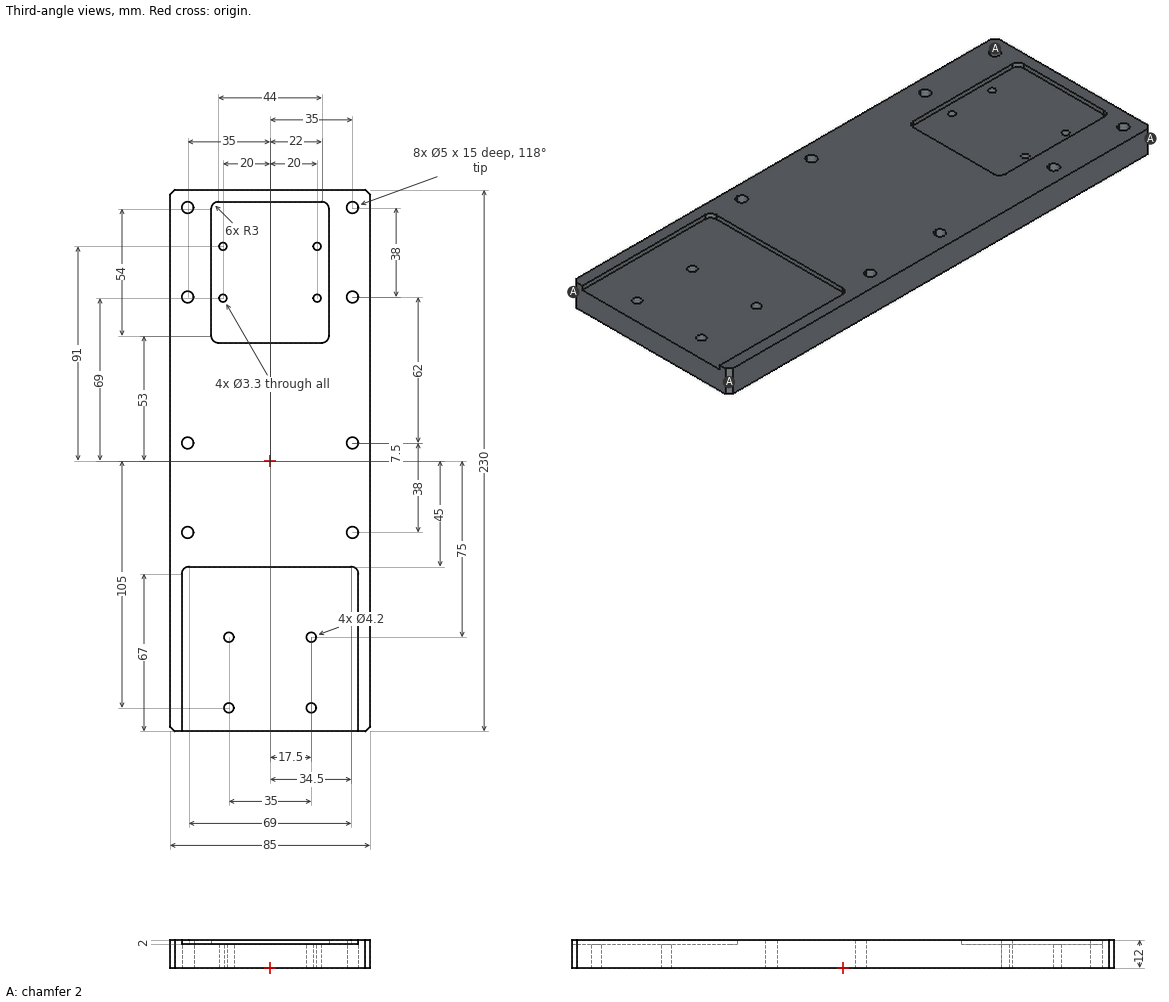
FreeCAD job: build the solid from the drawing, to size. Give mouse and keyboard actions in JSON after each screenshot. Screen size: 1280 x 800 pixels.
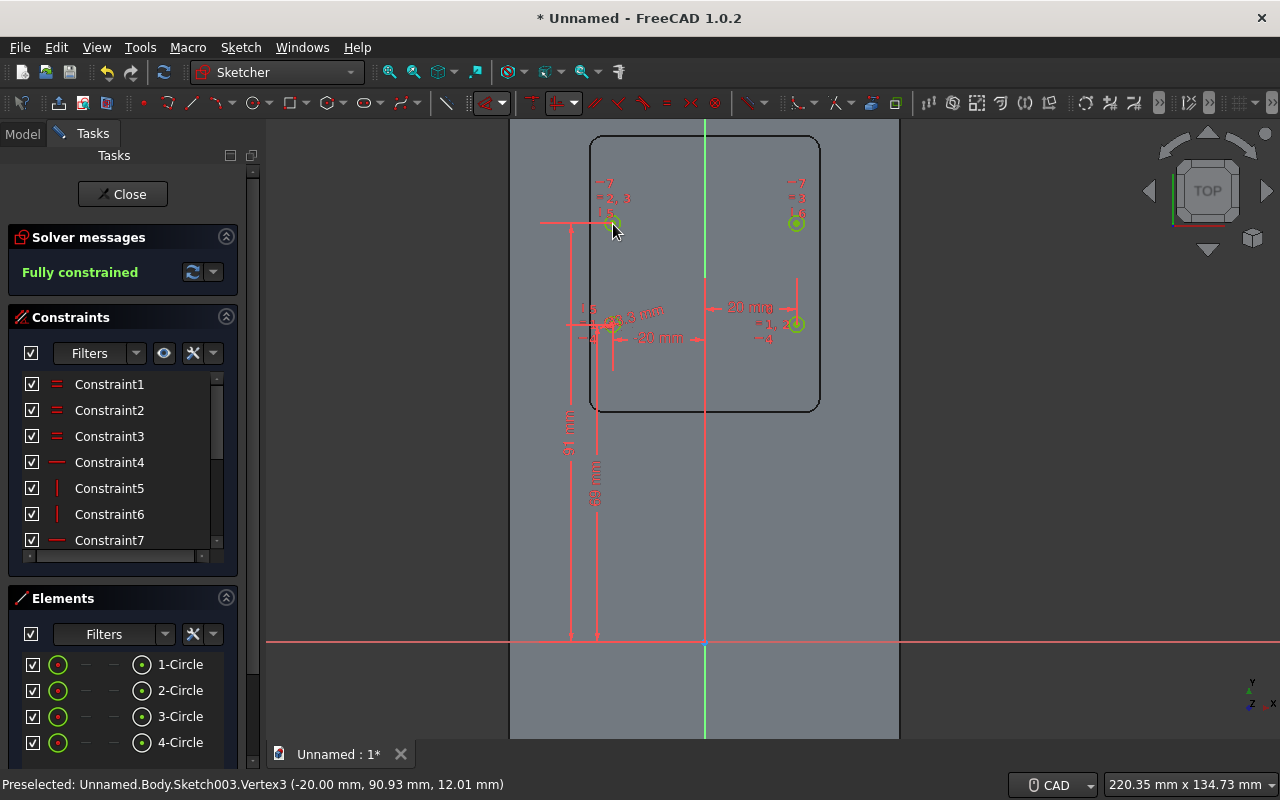
{"action": "left_click", "coordinate": [123, 194]}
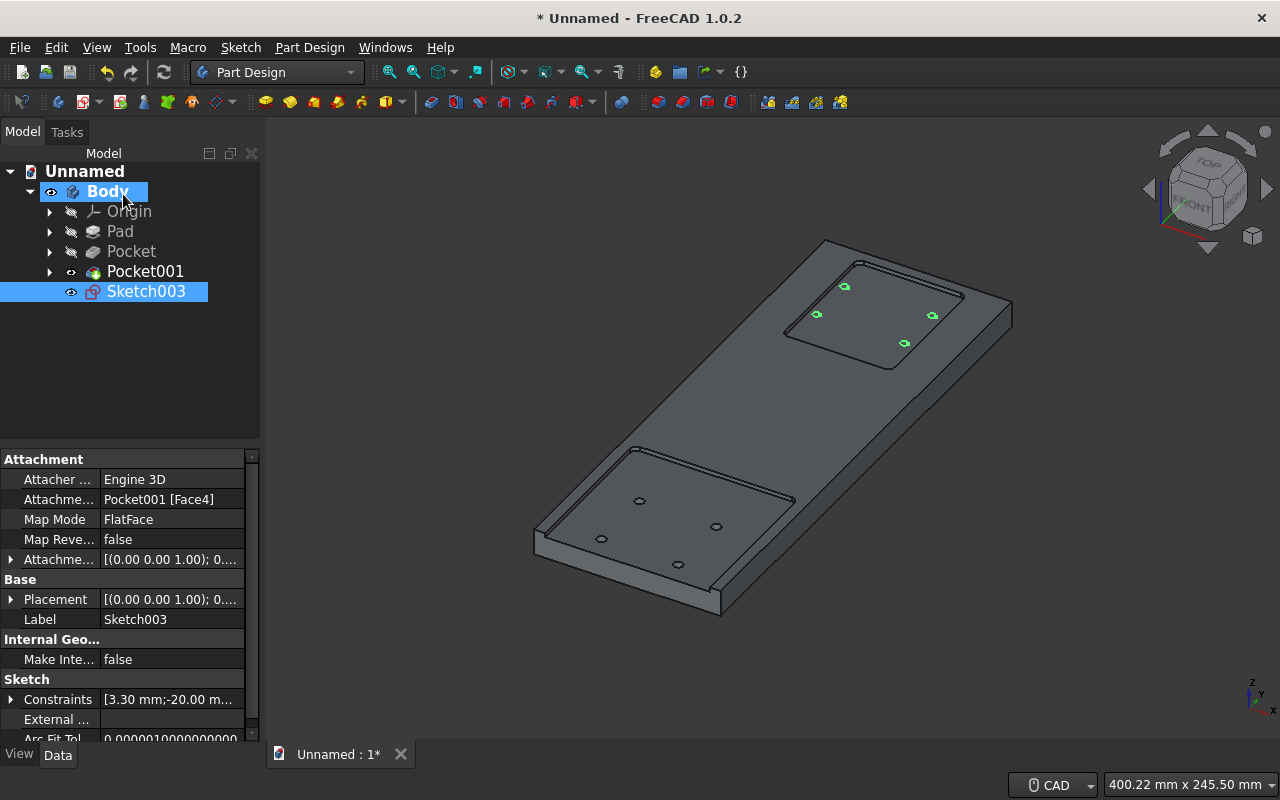
{"action": "left_click", "coordinate": [456, 102]}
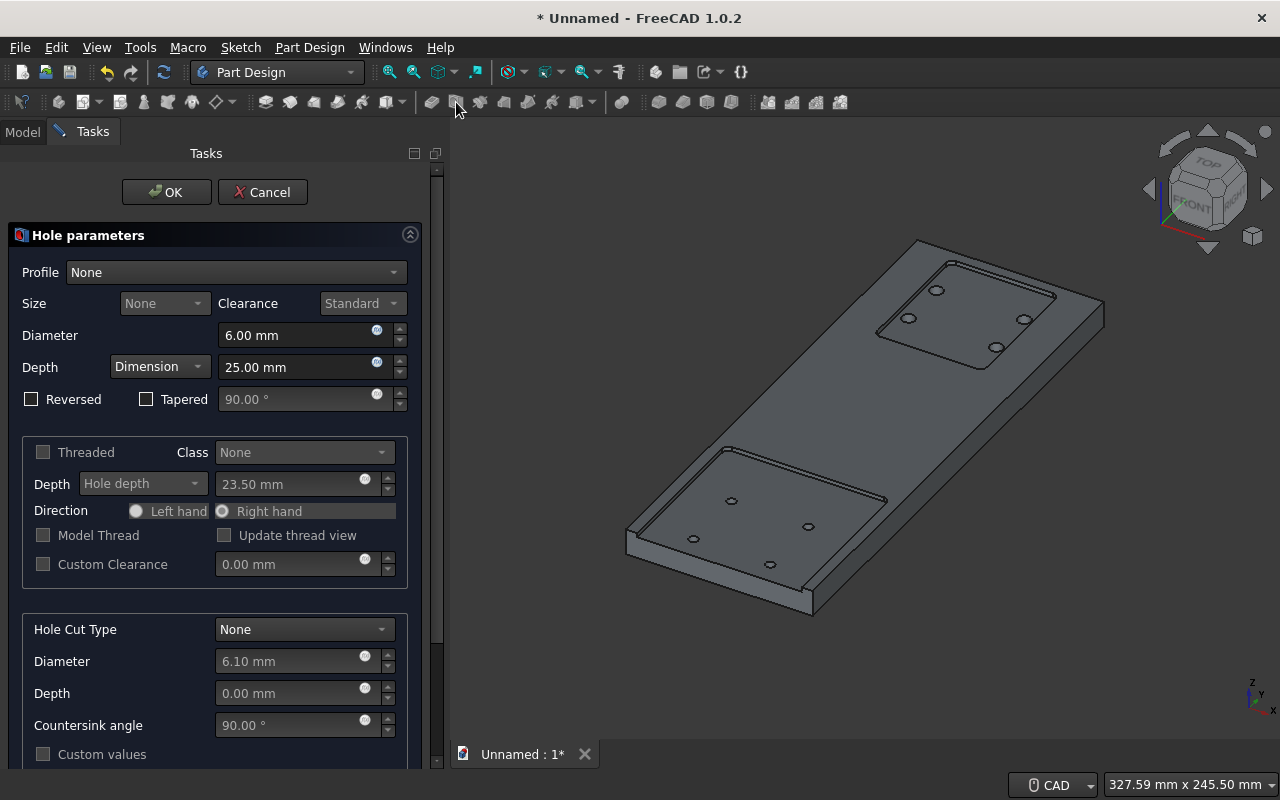
{"action": "triple_click", "coordinate": [305, 335]}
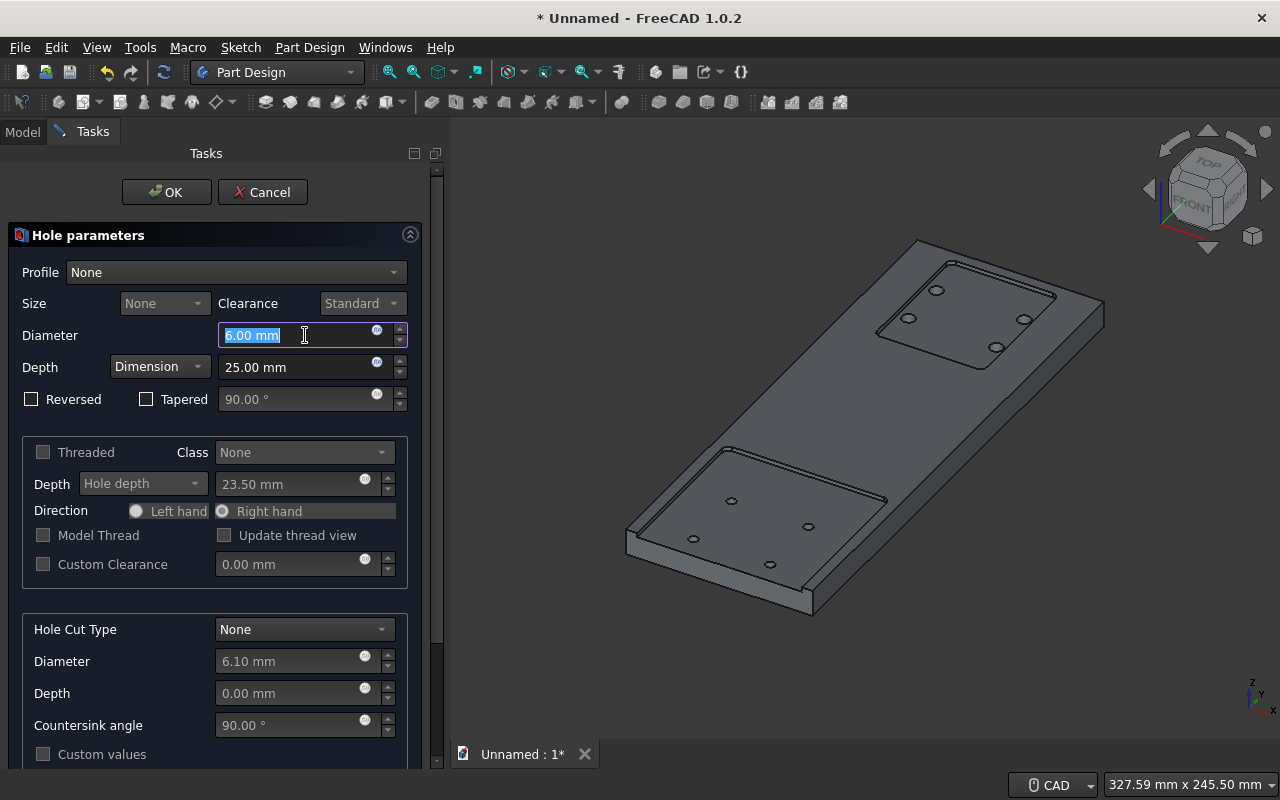
{"action": "type", "text": "3.3"}
{"action": "key", "text": "Tab"}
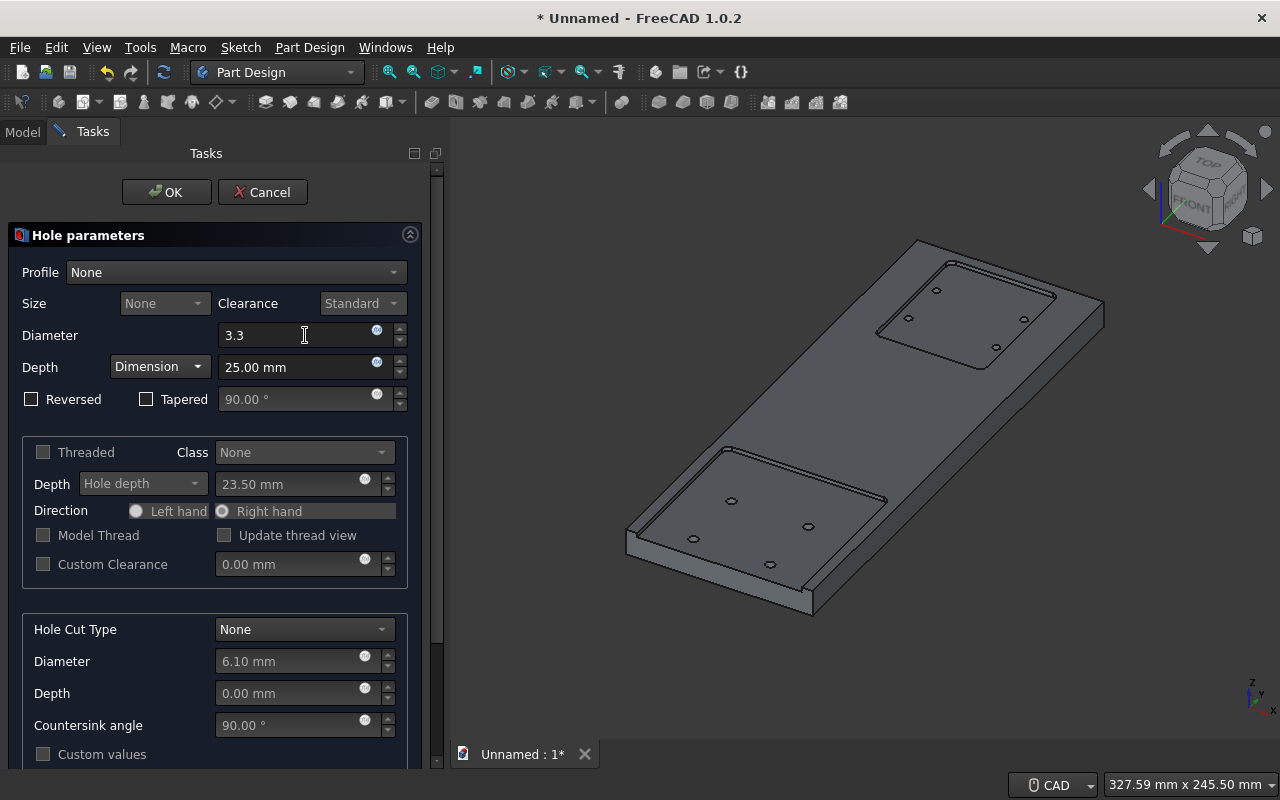
{"action": "left_click", "coordinate": [161, 366]}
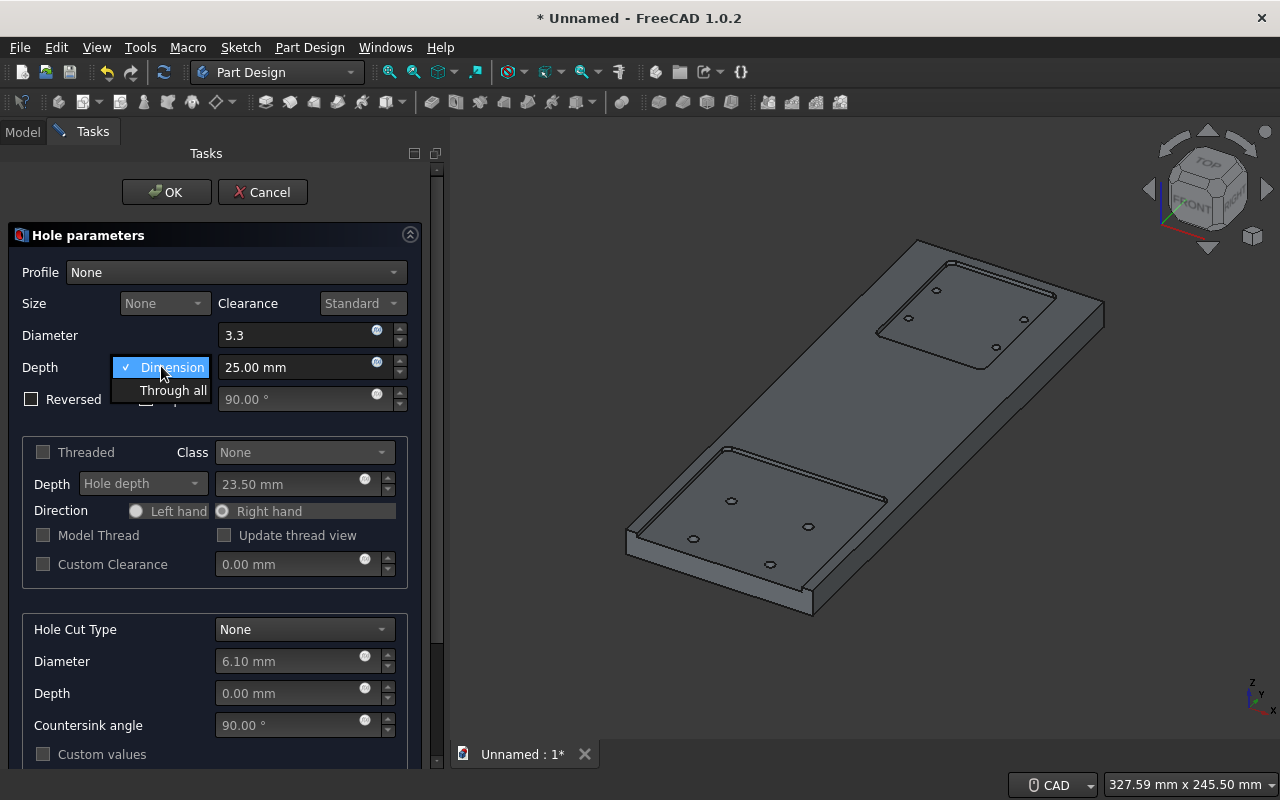
{"action": "left_click", "coordinate": [160, 390]}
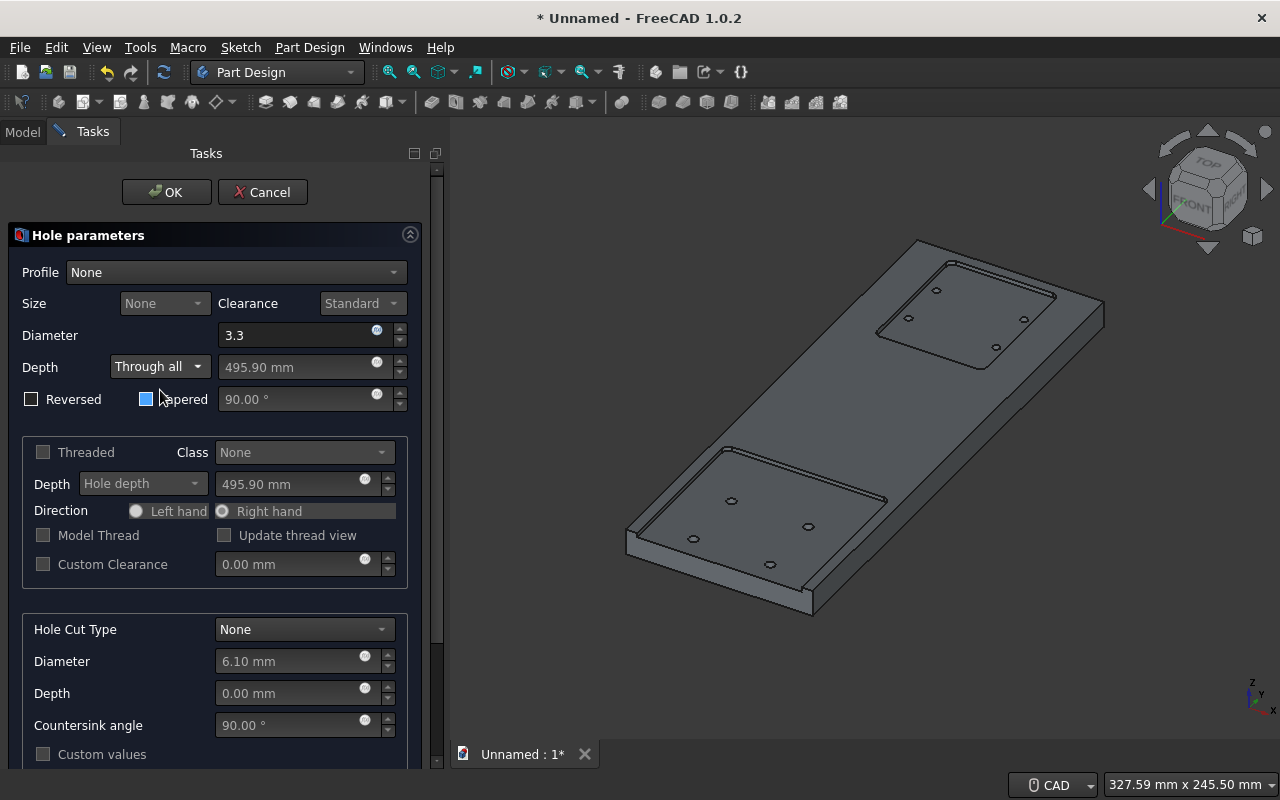
{"action": "left_click", "coordinate": [167, 192]}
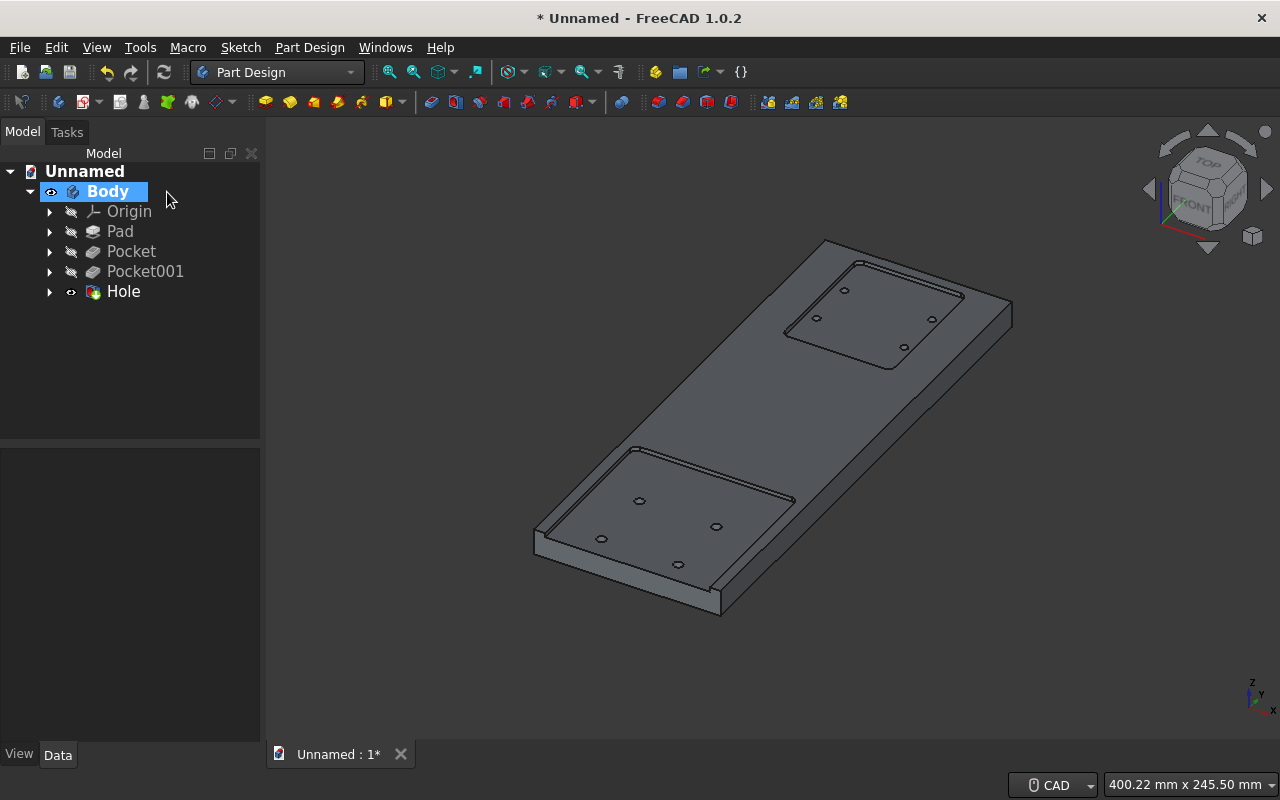
{"action": "left_click", "coordinate": [84, 102]}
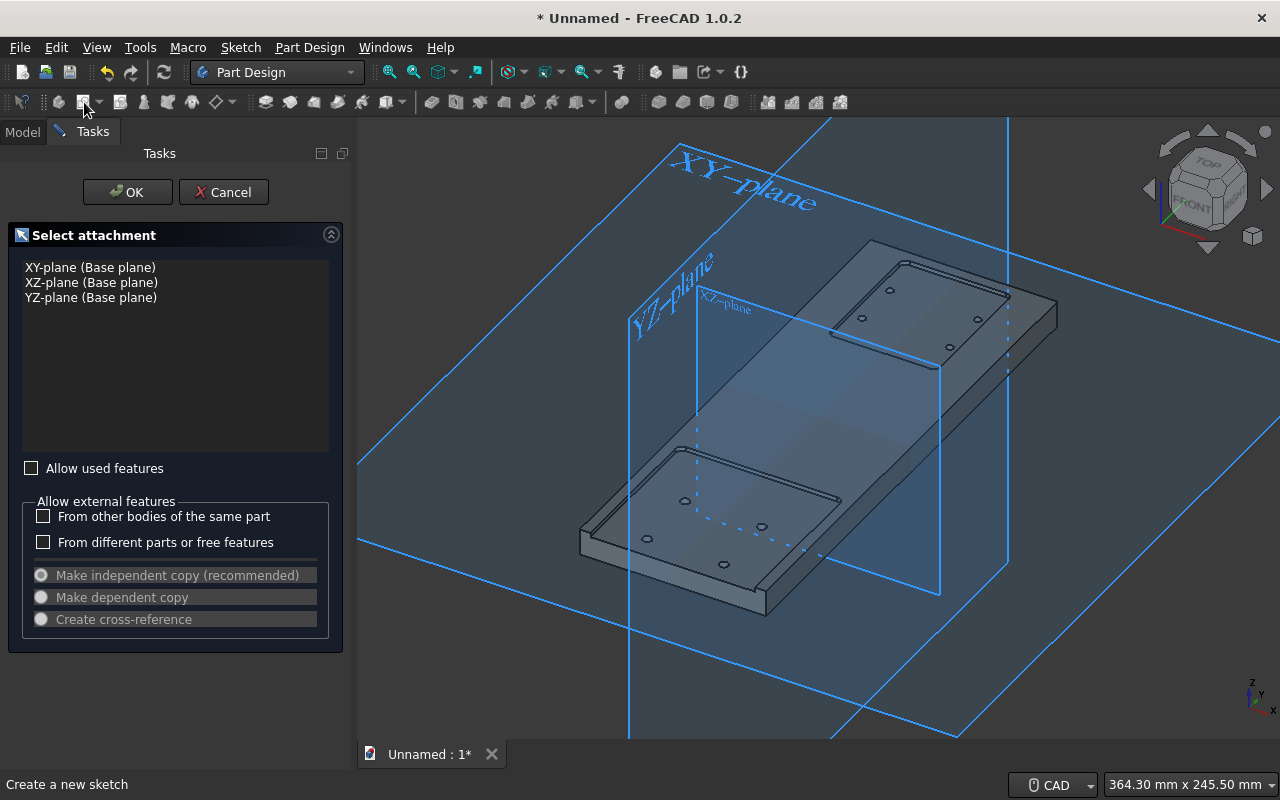
{"action": "left_click", "coordinate": [82, 268]}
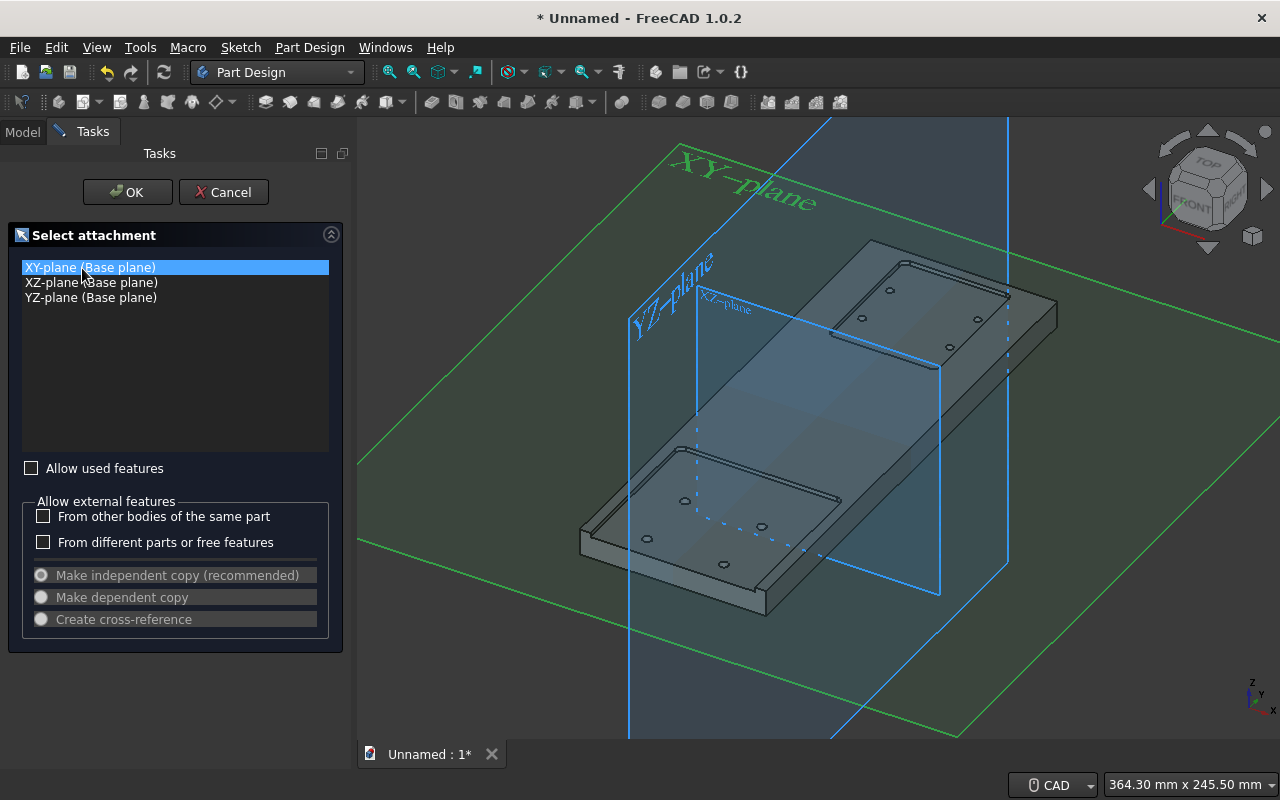
{"action": "left_click", "coordinate": [128, 192]}